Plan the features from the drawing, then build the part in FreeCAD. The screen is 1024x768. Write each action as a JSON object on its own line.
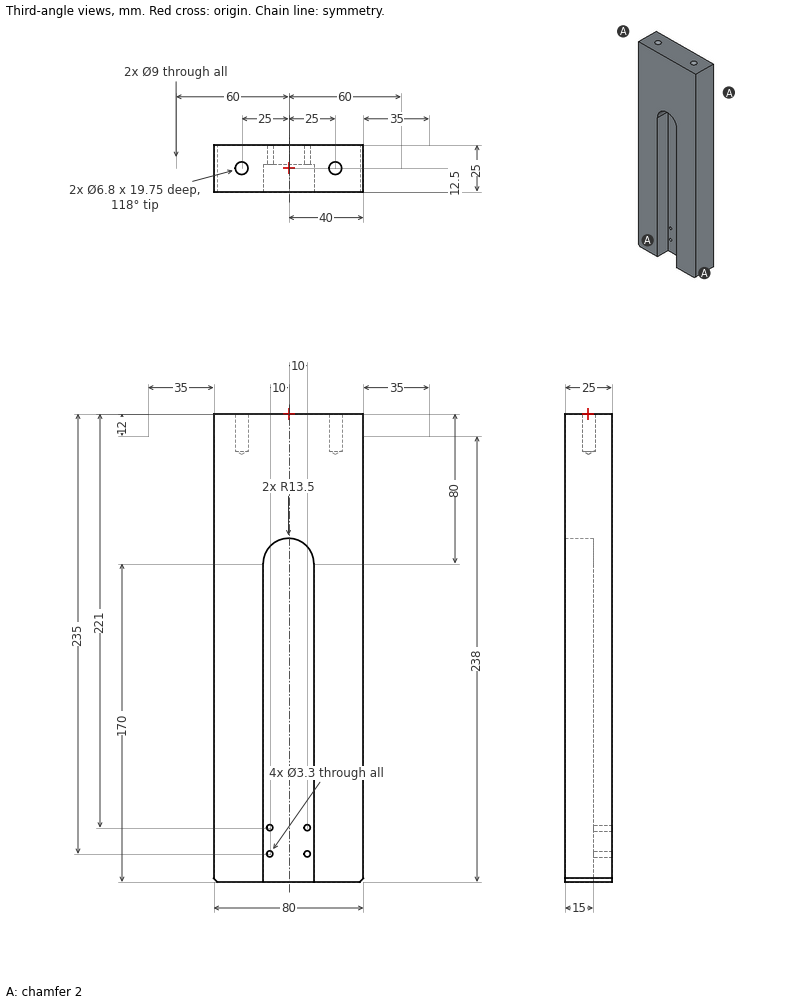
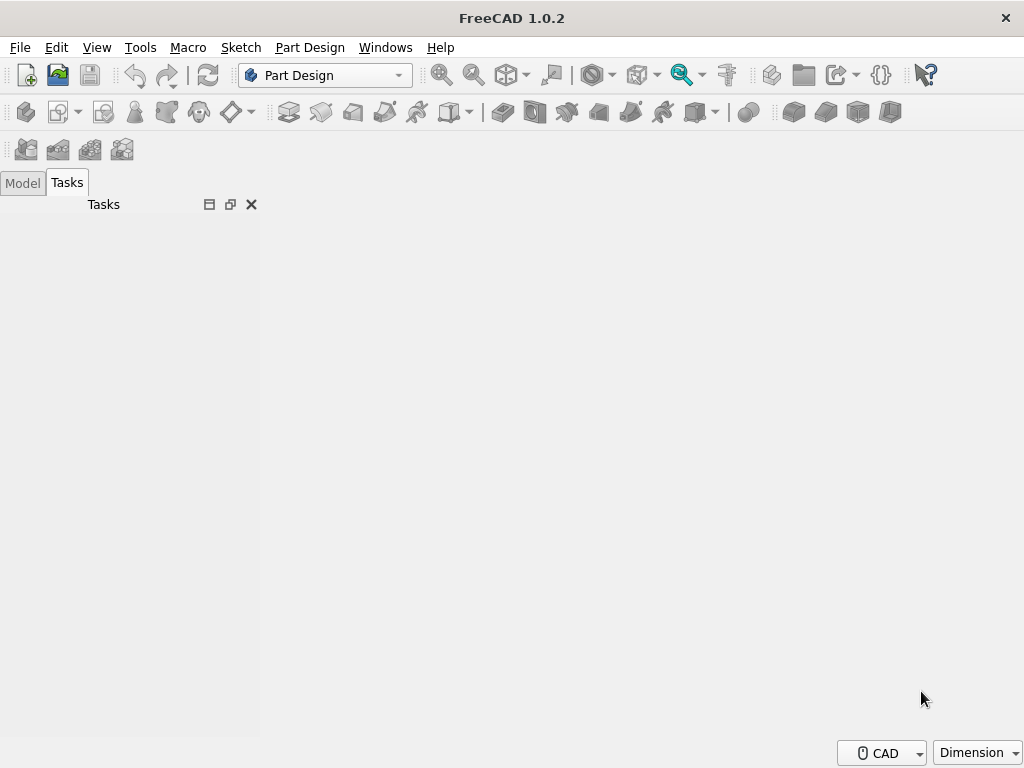
{"action": "left_click", "coordinate": [26, 76]}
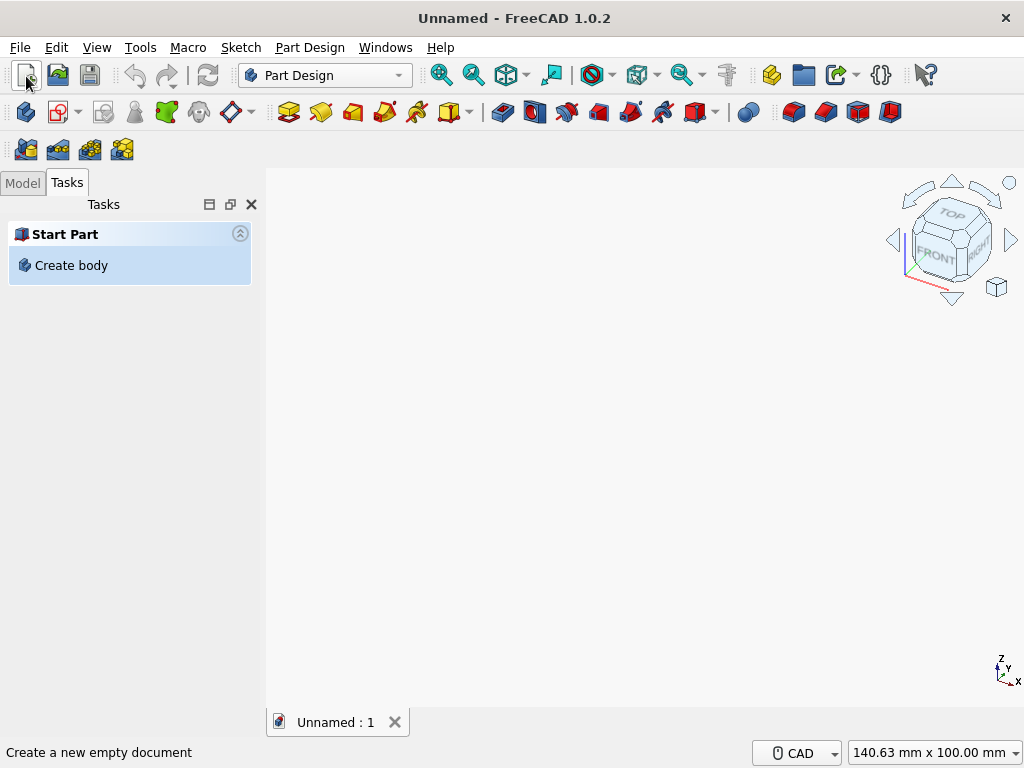
{"action": "left_click", "coordinate": [58, 112]}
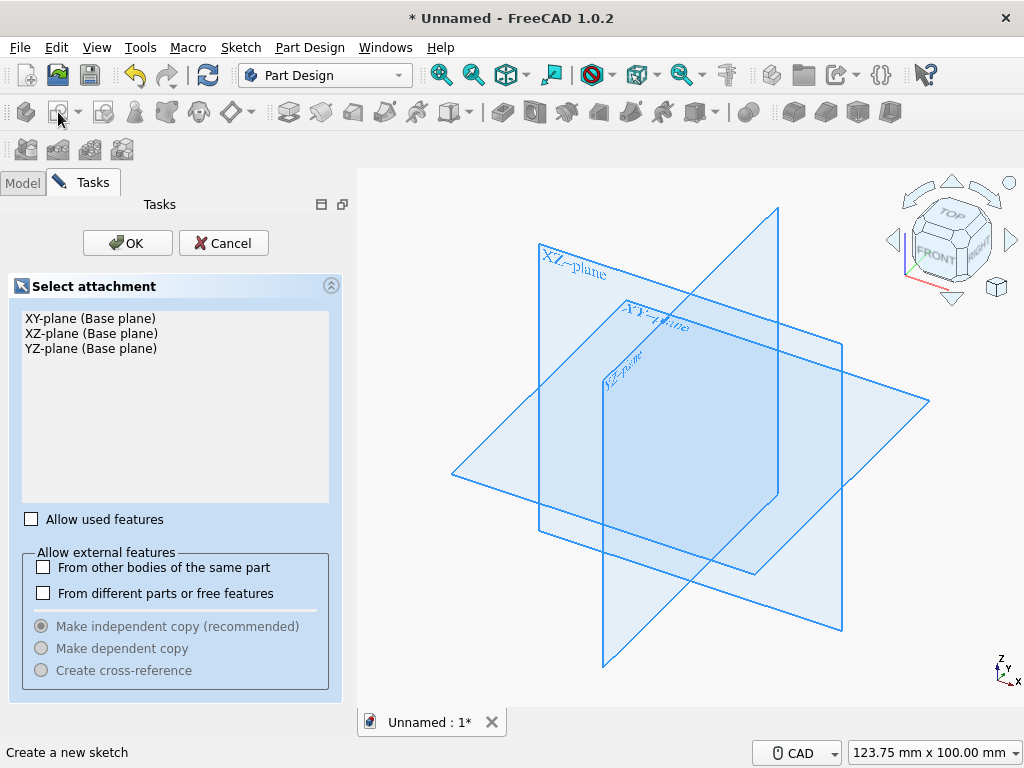
{"action": "left_click", "coordinate": [82, 334]}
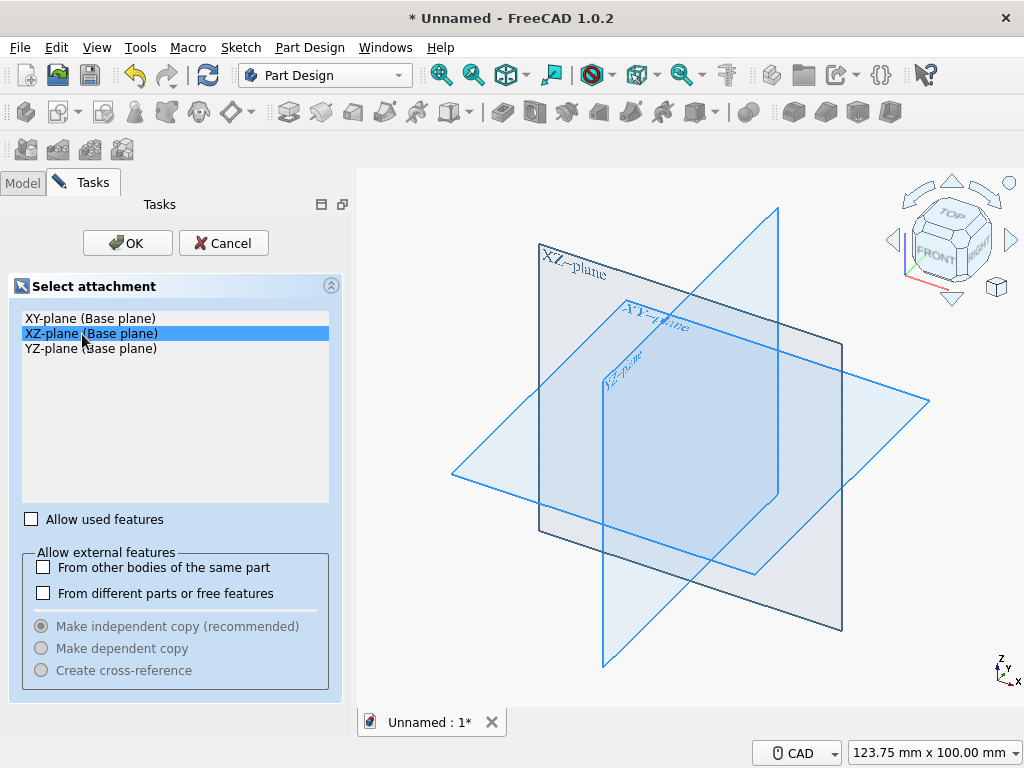
{"action": "left_click", "coordinate": [128, 243]}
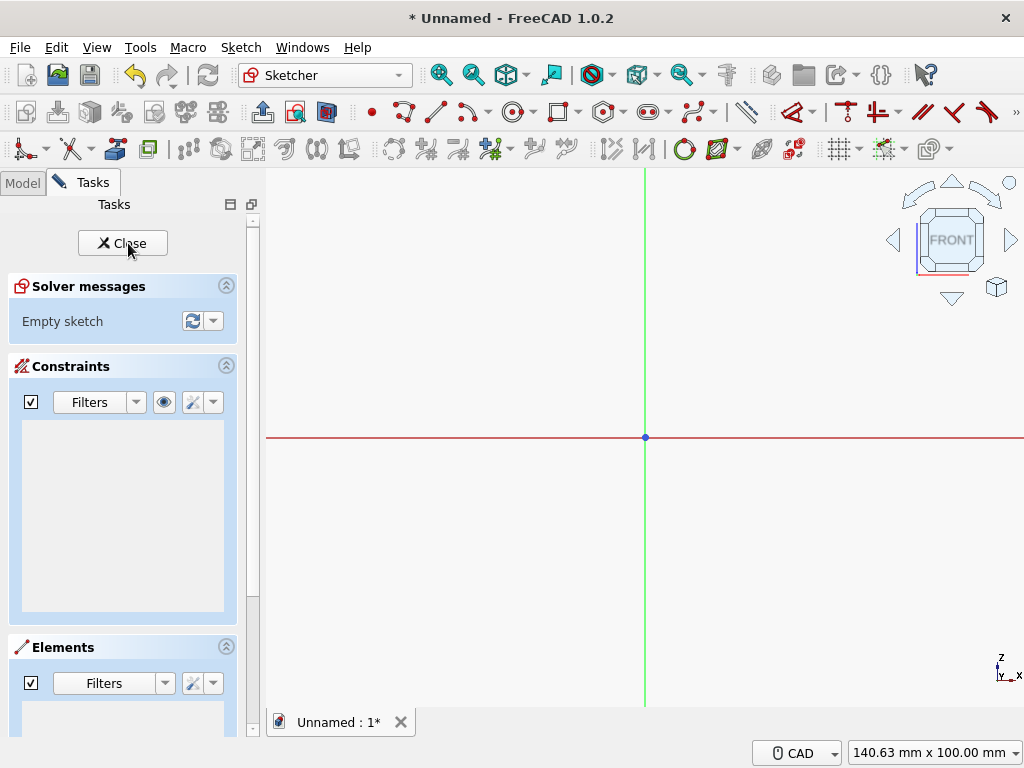
{"action": "scroll", "coordinate": [554, 217], "scroll_direction": "down", "scroll_amount": 7}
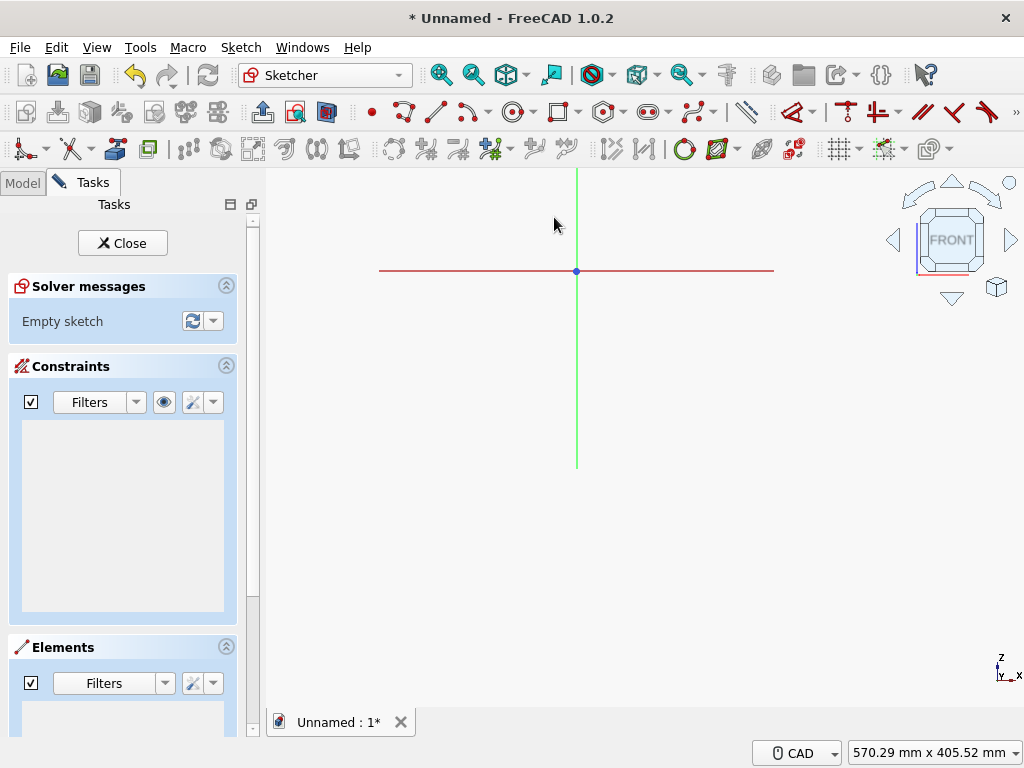
{"action": "left_click", "coordinate": [404, 112]}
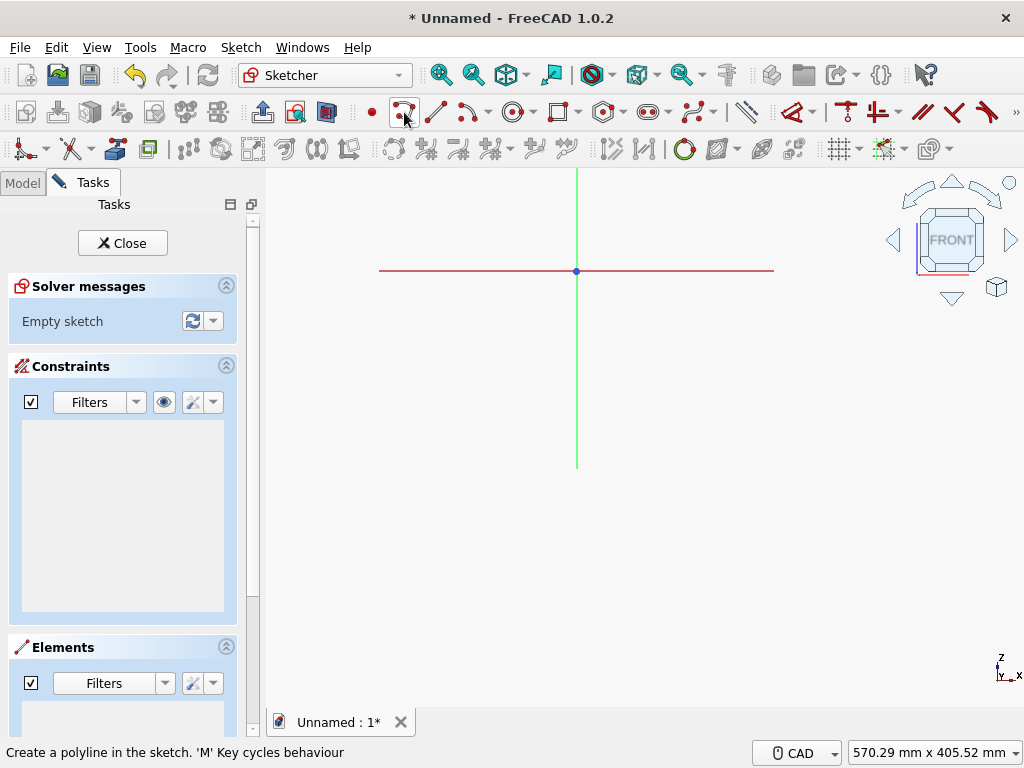
{"action": "left_click", "coordinate": [630, 287]}
{"action": "left_click", "coordinate": [630, 604]}
{"action": "left_click", "coordinate": [524, 604]}
{"action": "left_click", "coordinate": [524, 287]}
{"action": "left_click", "coordinate": [477, 287]}
{"action": "left_click", "coordinate": [477, 271]}
{"action": "left_click", "coordinate": [676, 280]}
{"action": "left_click", "coordinate": [676, 287]}
{"action": "left_click", "coordinate": [630, 288]}
{"action": "key", "text": "Escape"}
{"action": "key", "text": "Escape"}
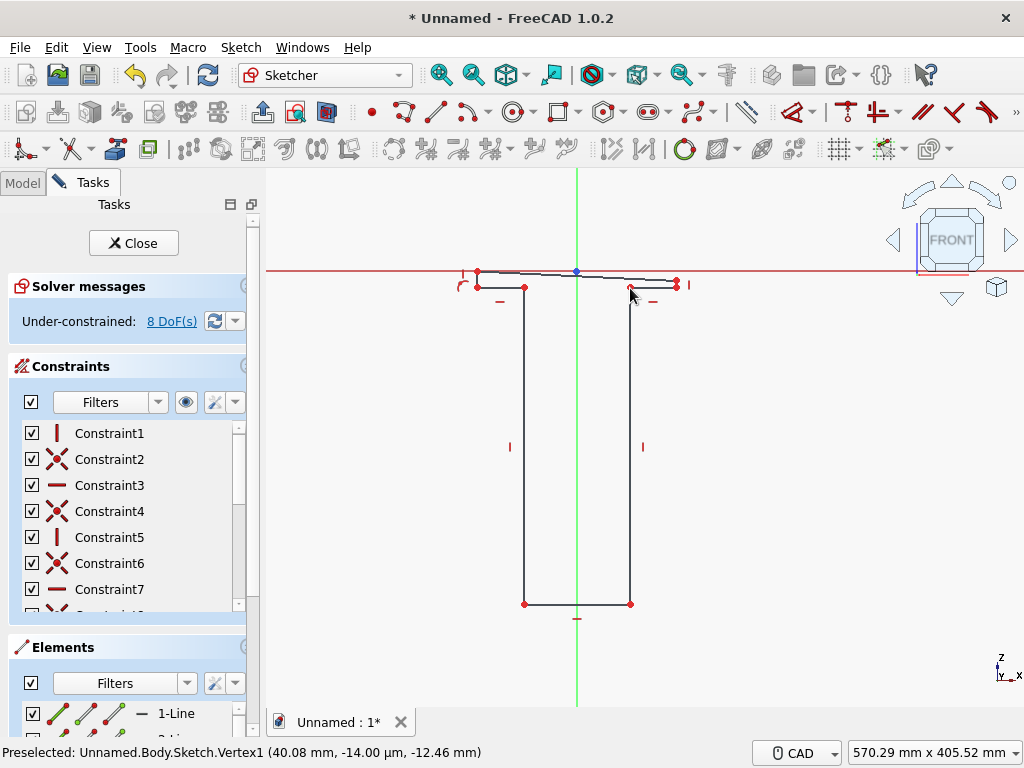
{"action": "left_click", "coordinate": [537, 274]}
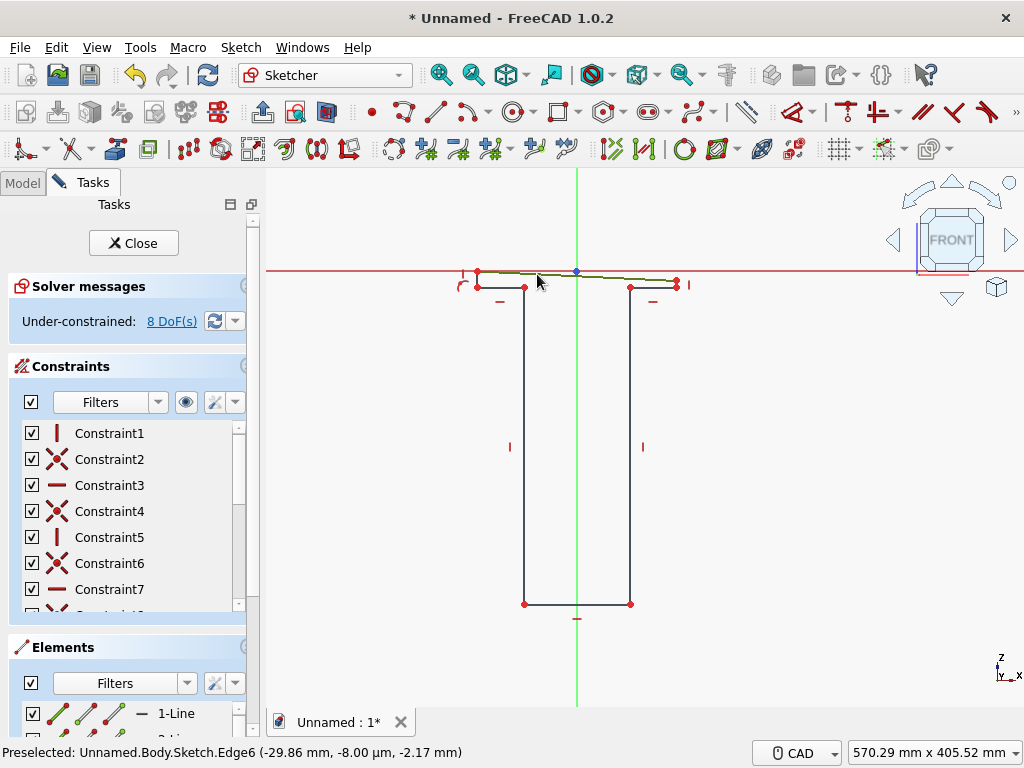
{"action": "key", "text": "h"}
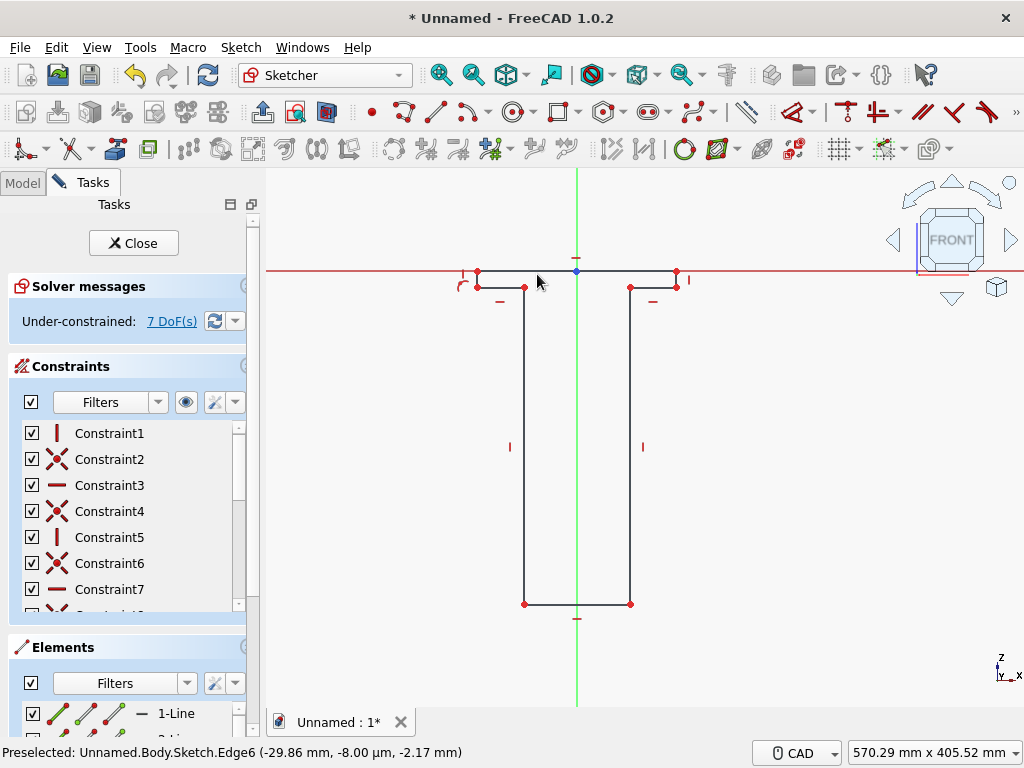
{"action": "left_click", "coordinate": [630, 288]}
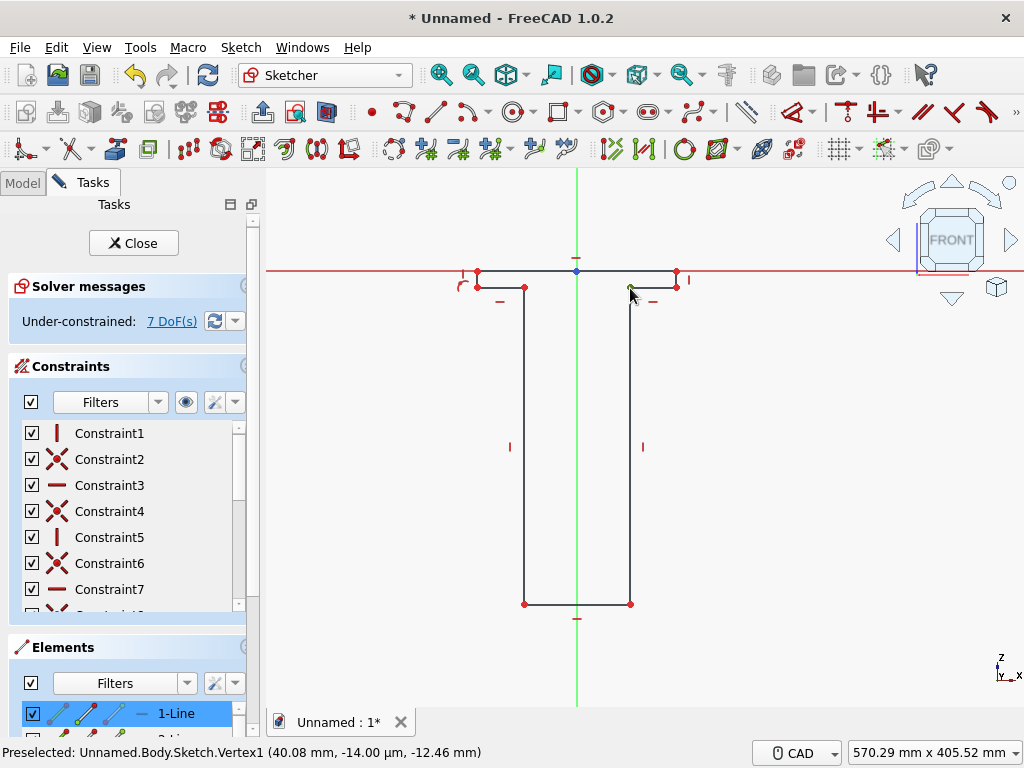
{"action": "left_click", "coordinate": [524, 288]}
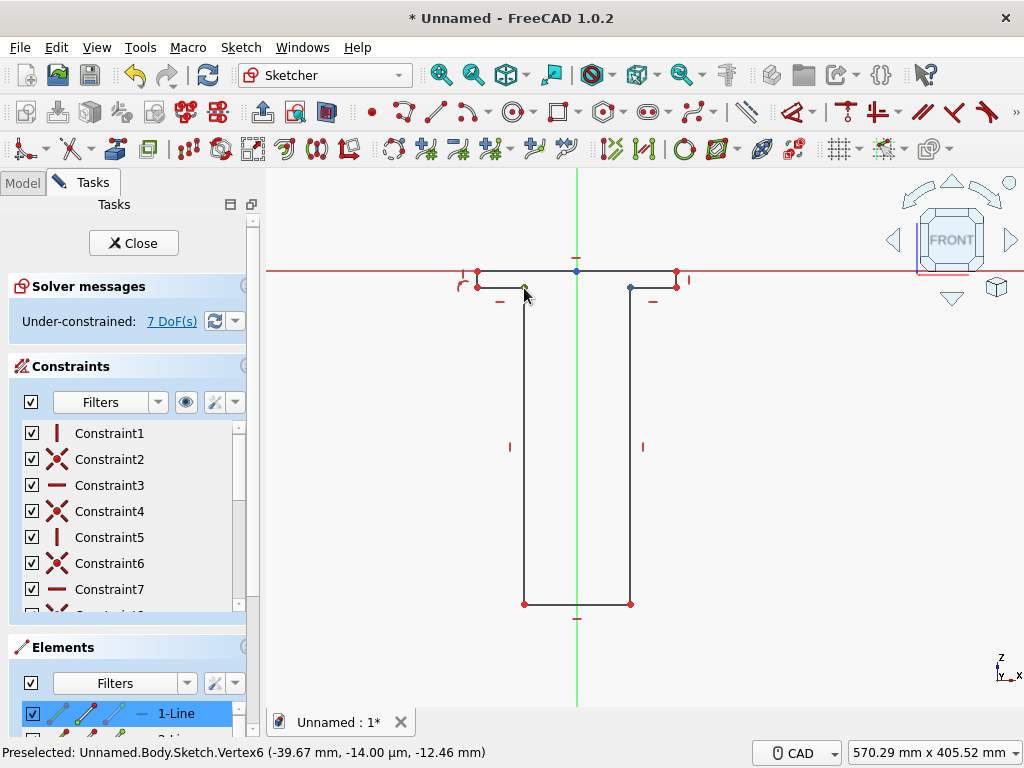
{"action": "left_click", "coordinate": [577, 644]}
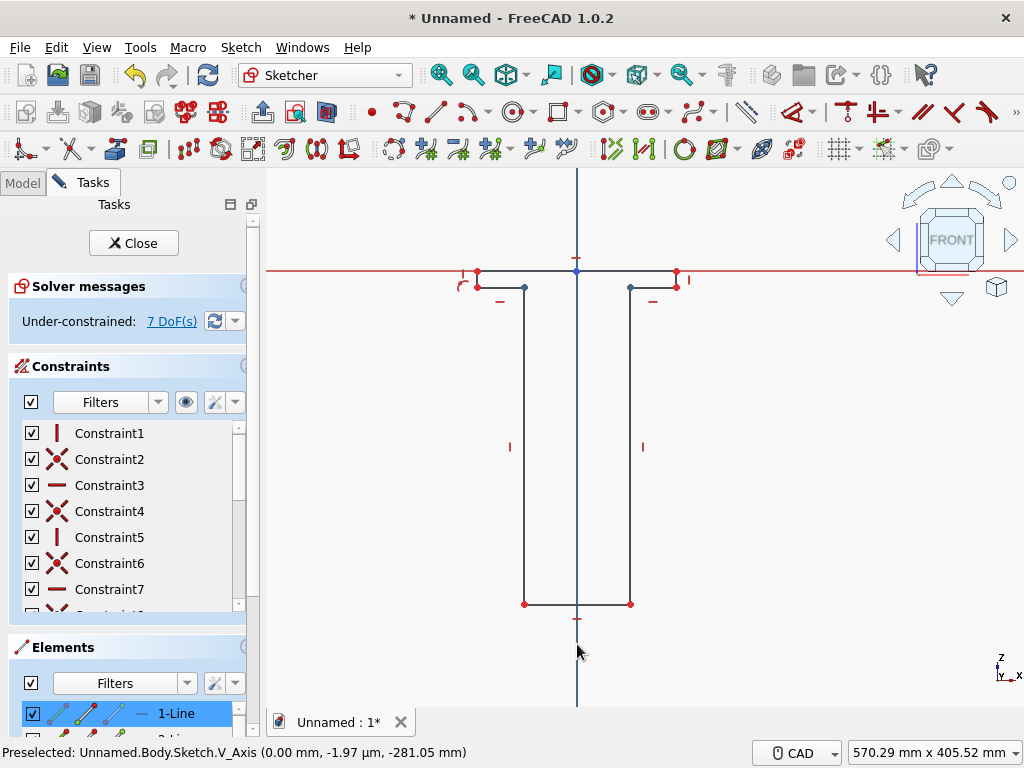
{"action": "key", "text": "s"}